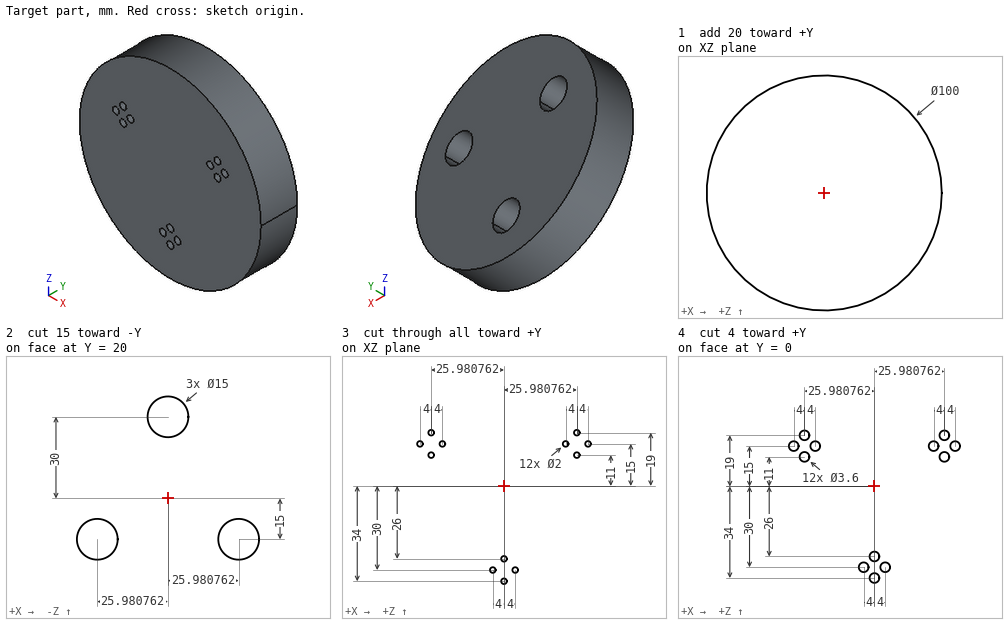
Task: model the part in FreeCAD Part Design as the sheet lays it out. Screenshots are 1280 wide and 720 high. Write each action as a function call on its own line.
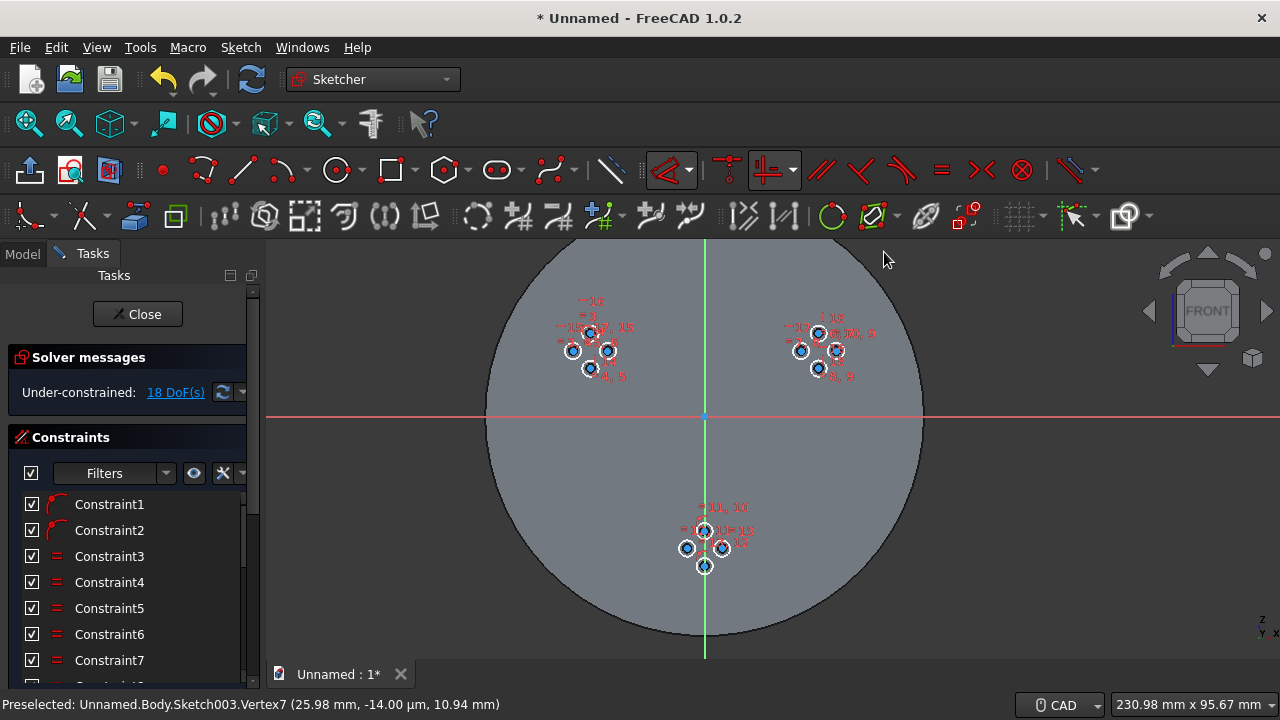
click(588, 371)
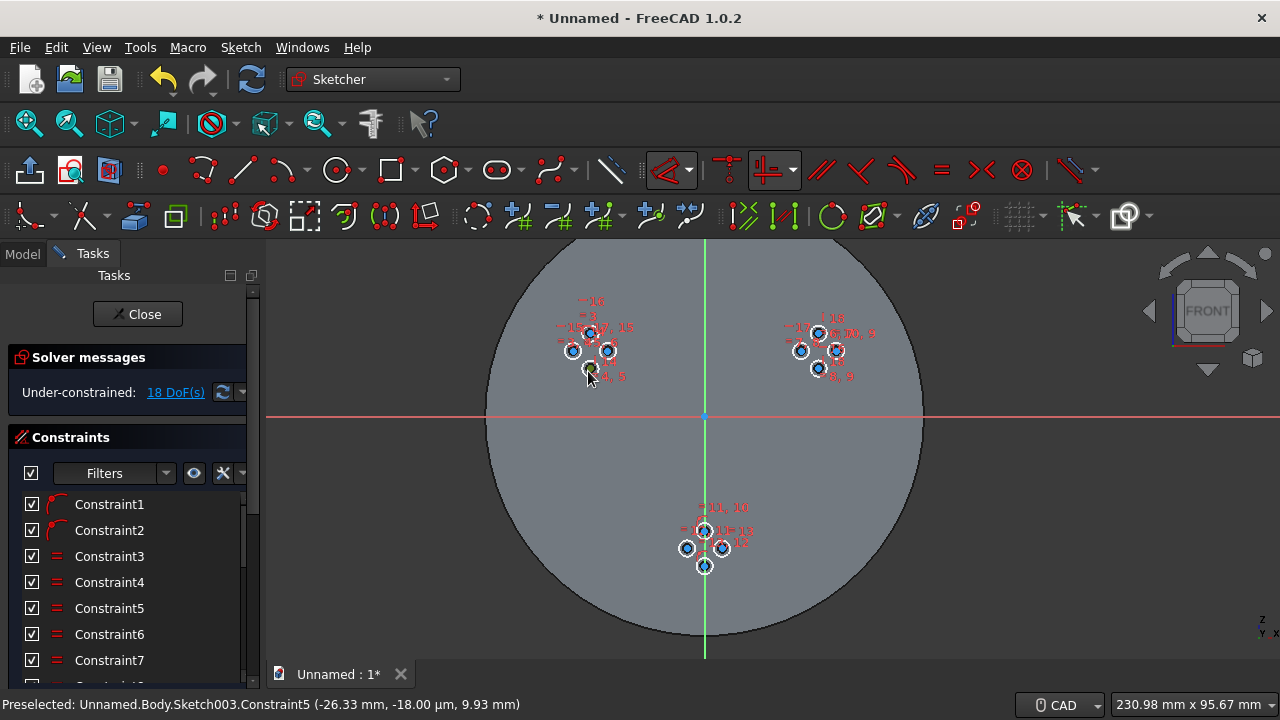
scroll(819, 369, up, 4)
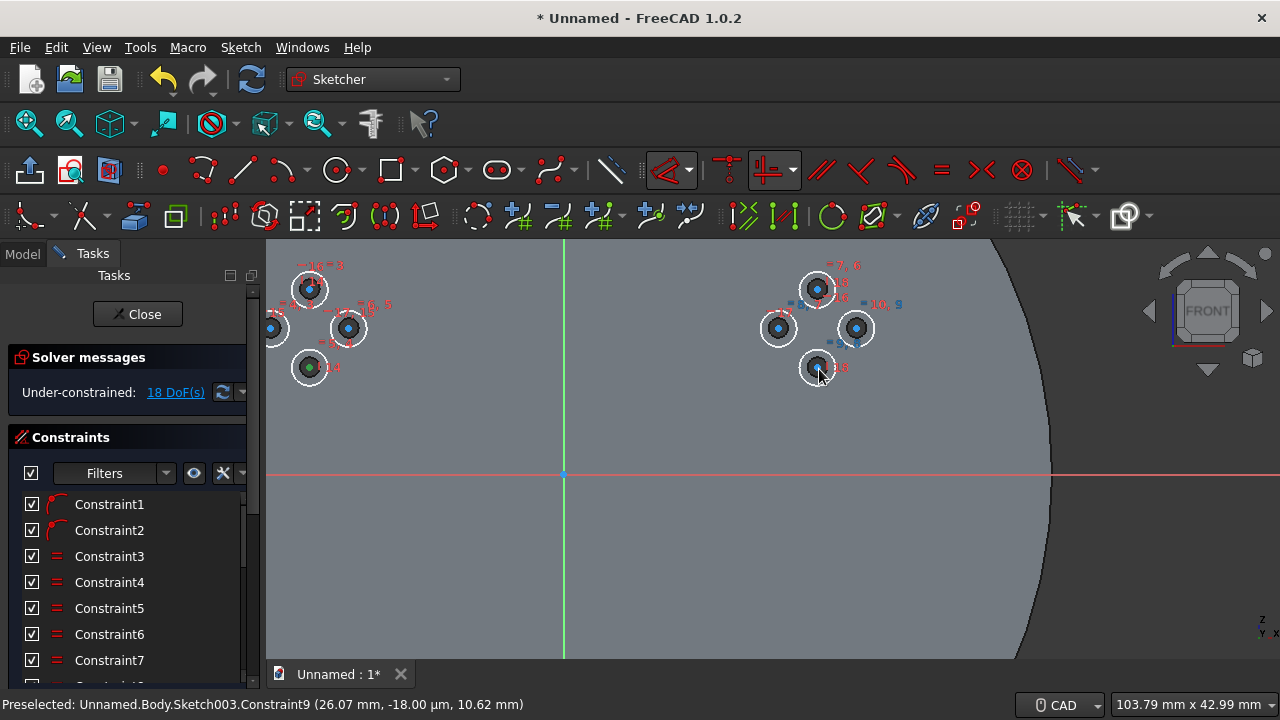
click(818, 368)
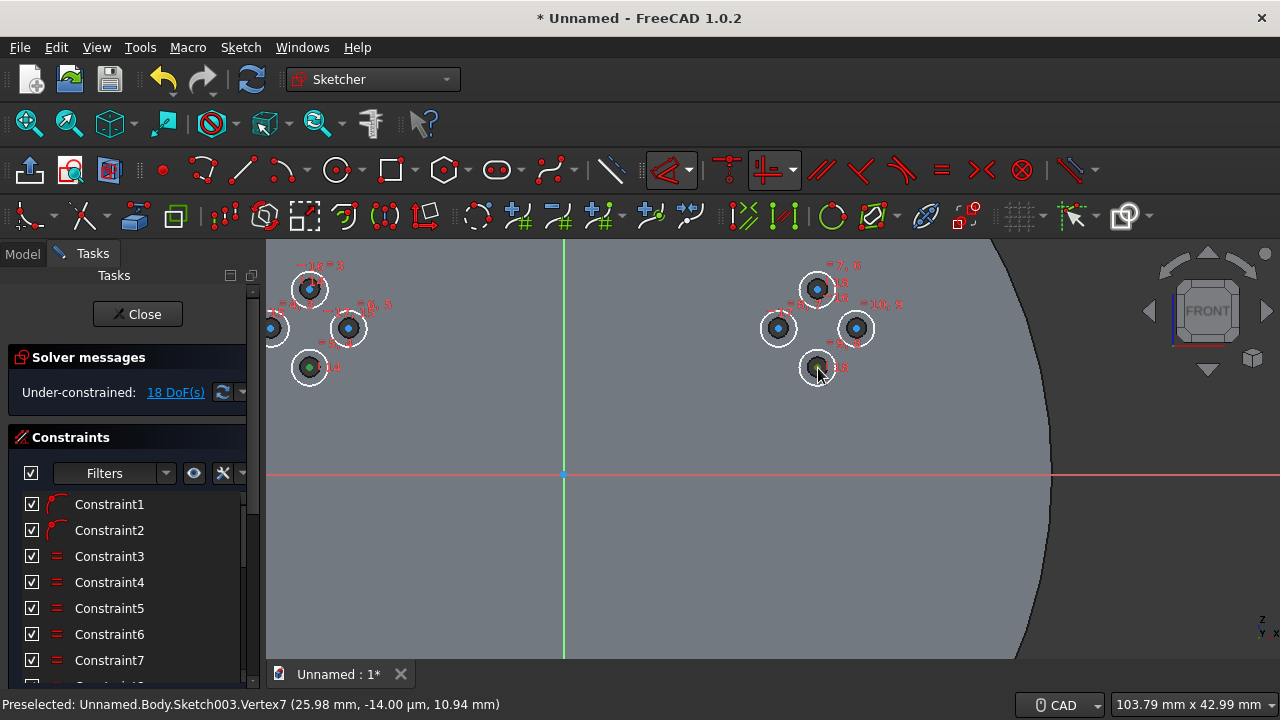
click(796, 170)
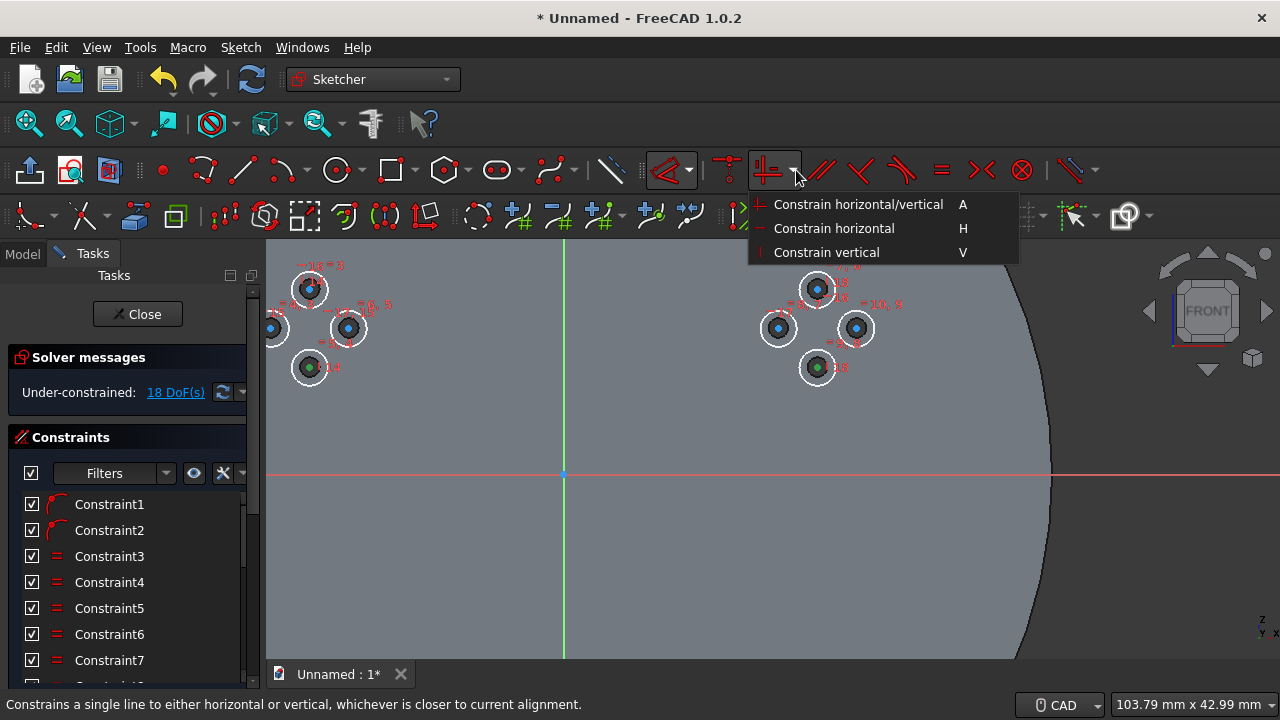
click(884, 228)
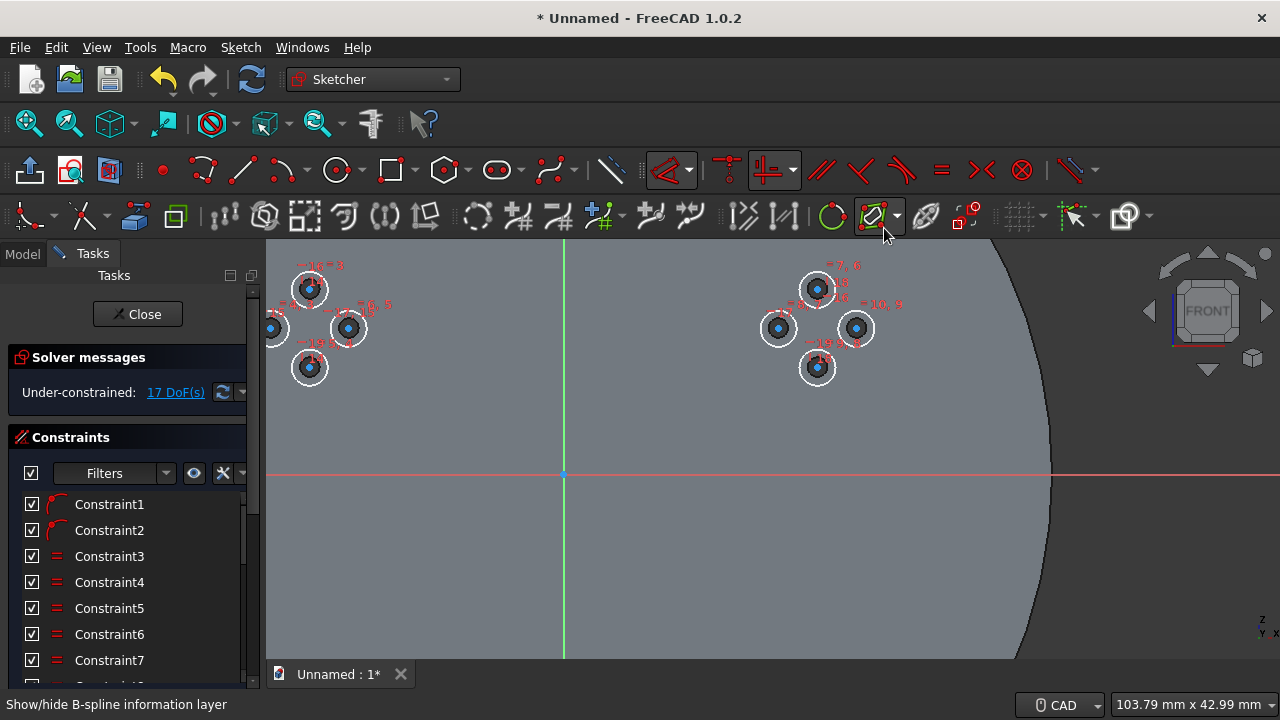
click(779, 329)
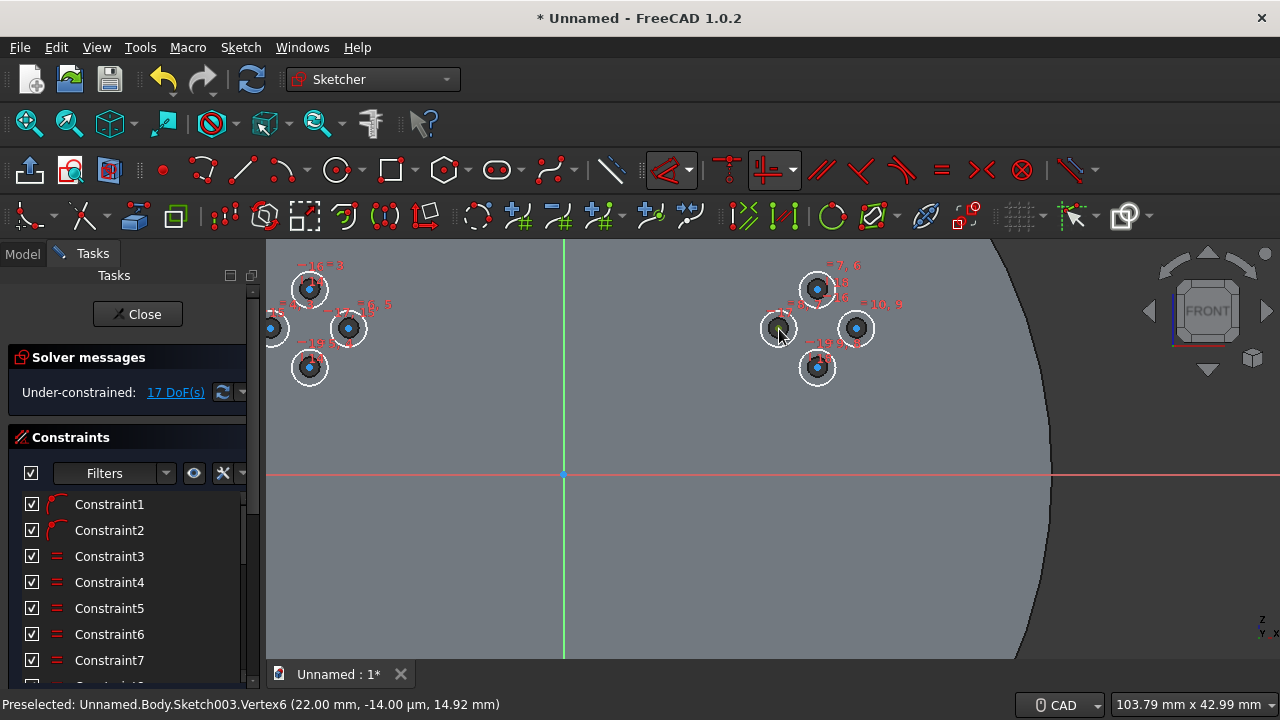
click(856, 329)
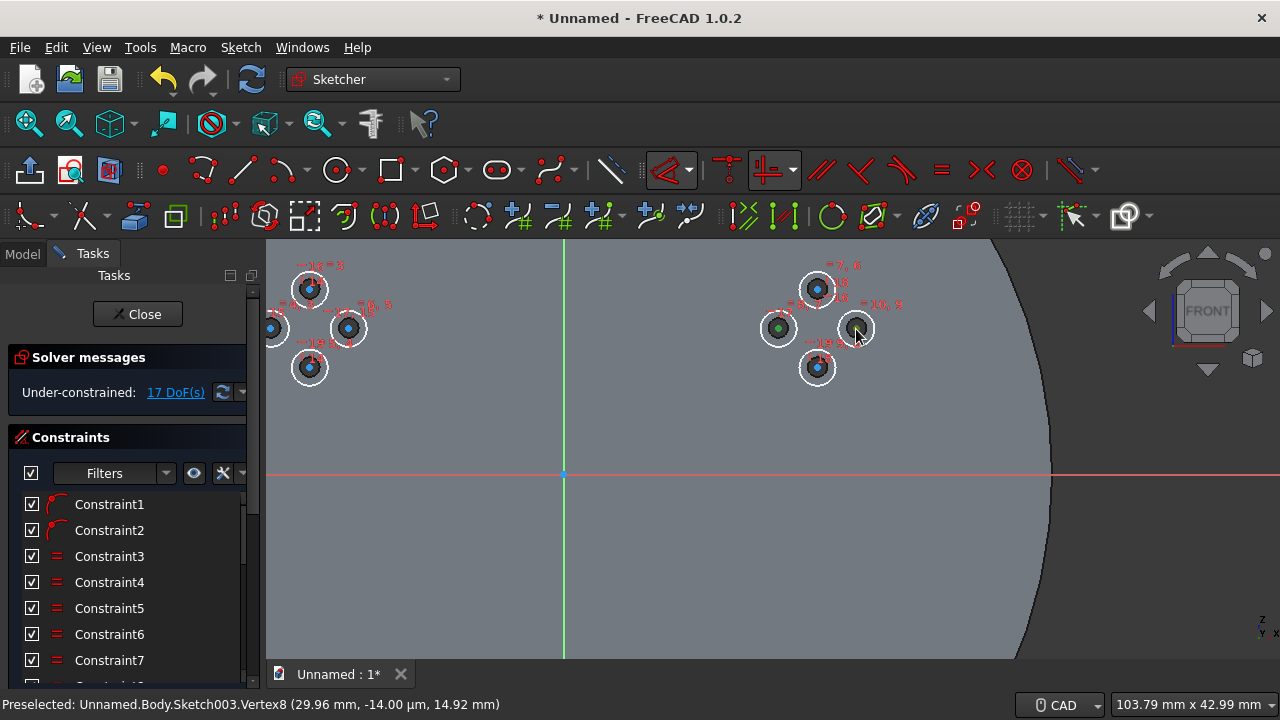
click(796, 170)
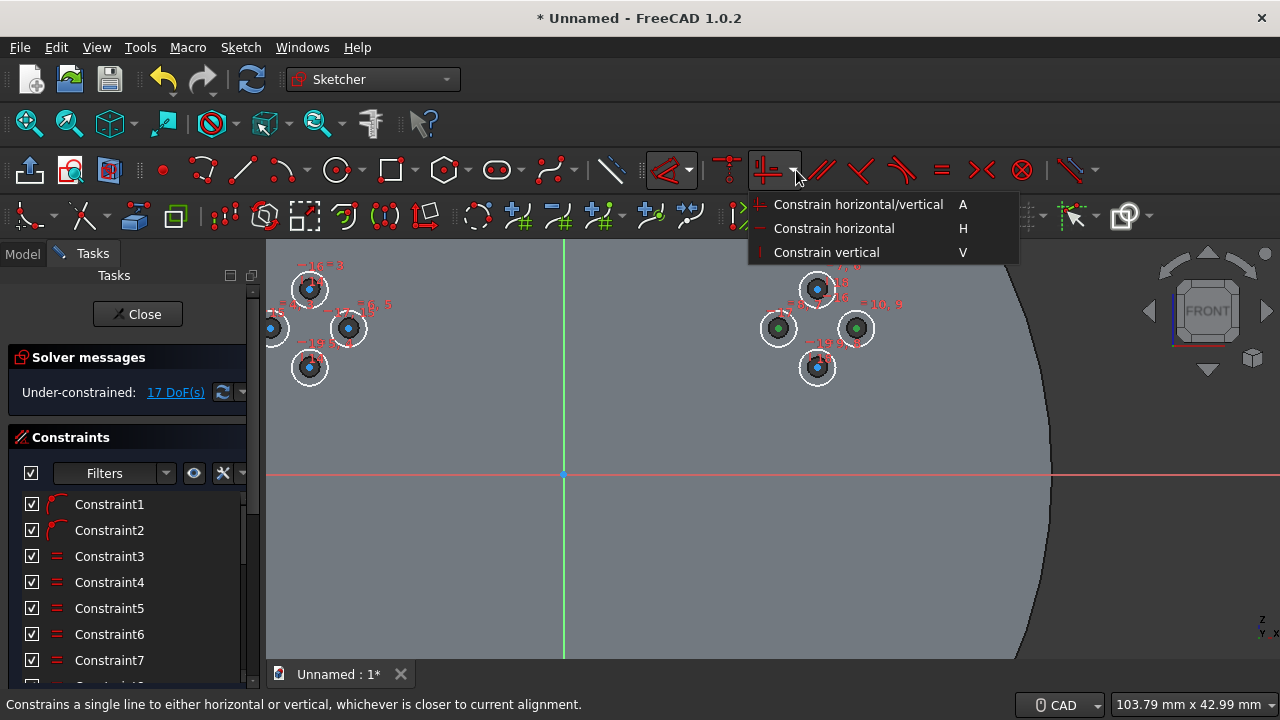
click(884, 228)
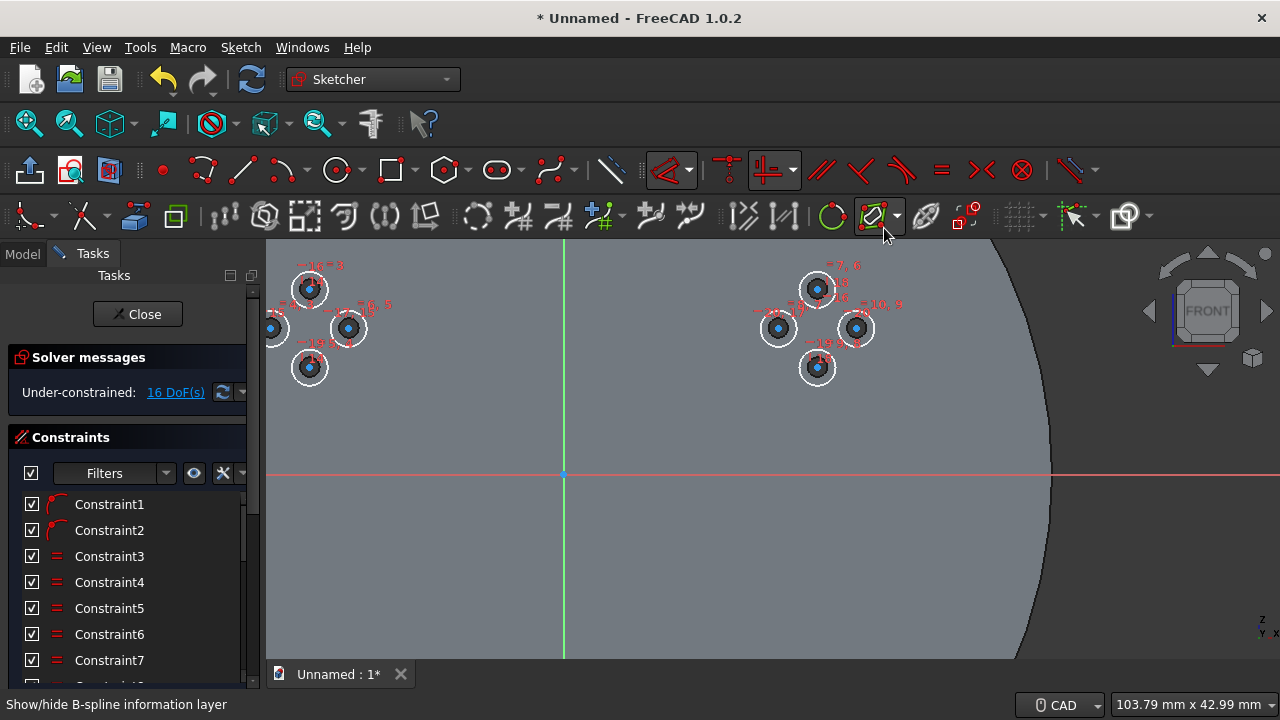
scroll(819, 368, down, 4)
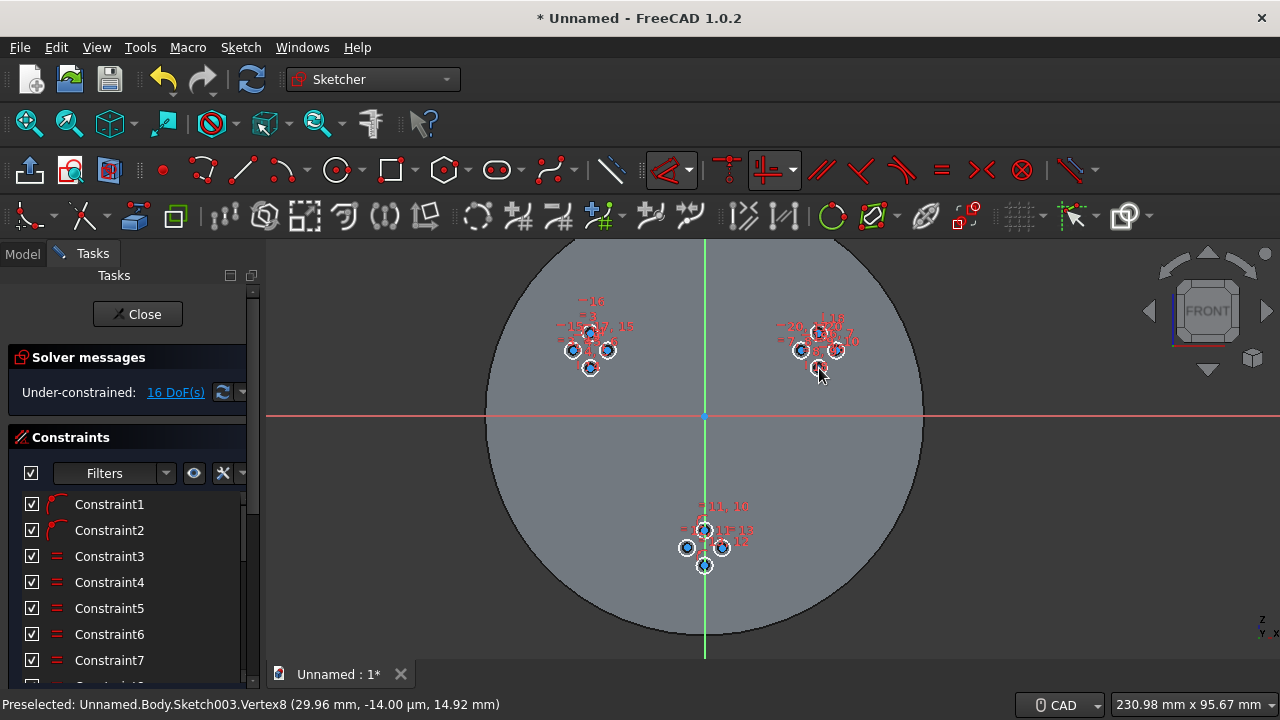
click(687, 548)